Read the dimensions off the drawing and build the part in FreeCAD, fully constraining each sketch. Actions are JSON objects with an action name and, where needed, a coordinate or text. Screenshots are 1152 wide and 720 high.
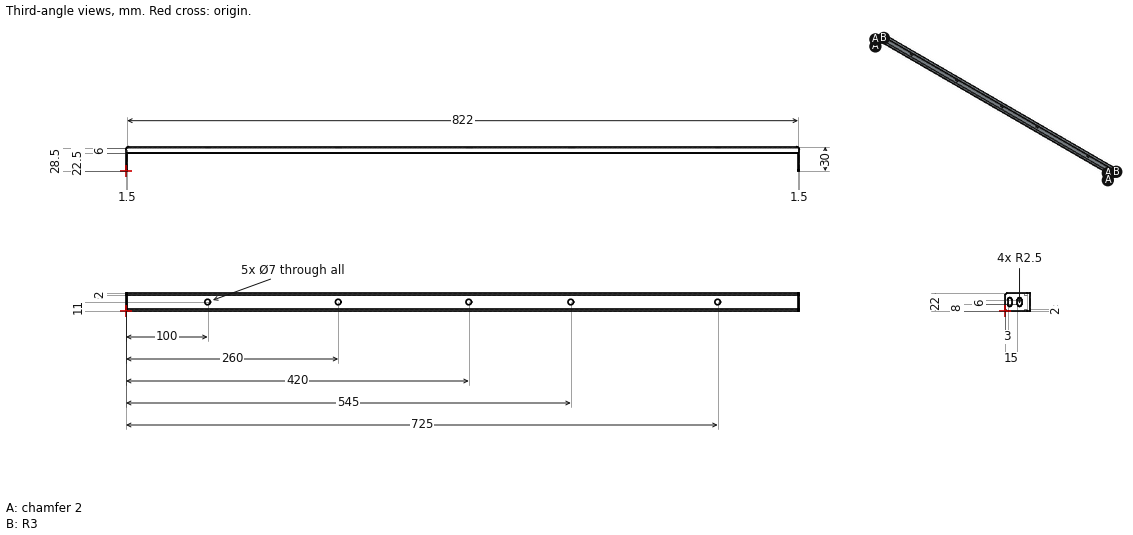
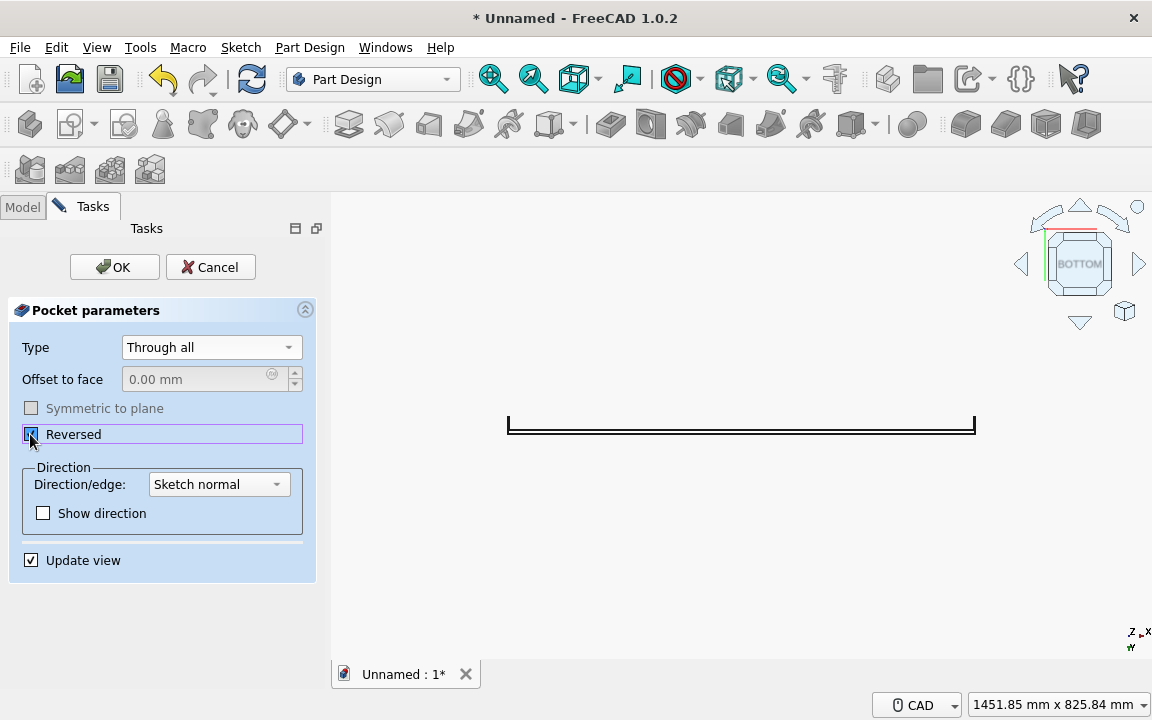
{"action": "left_click", "coordinate": [115, 267]}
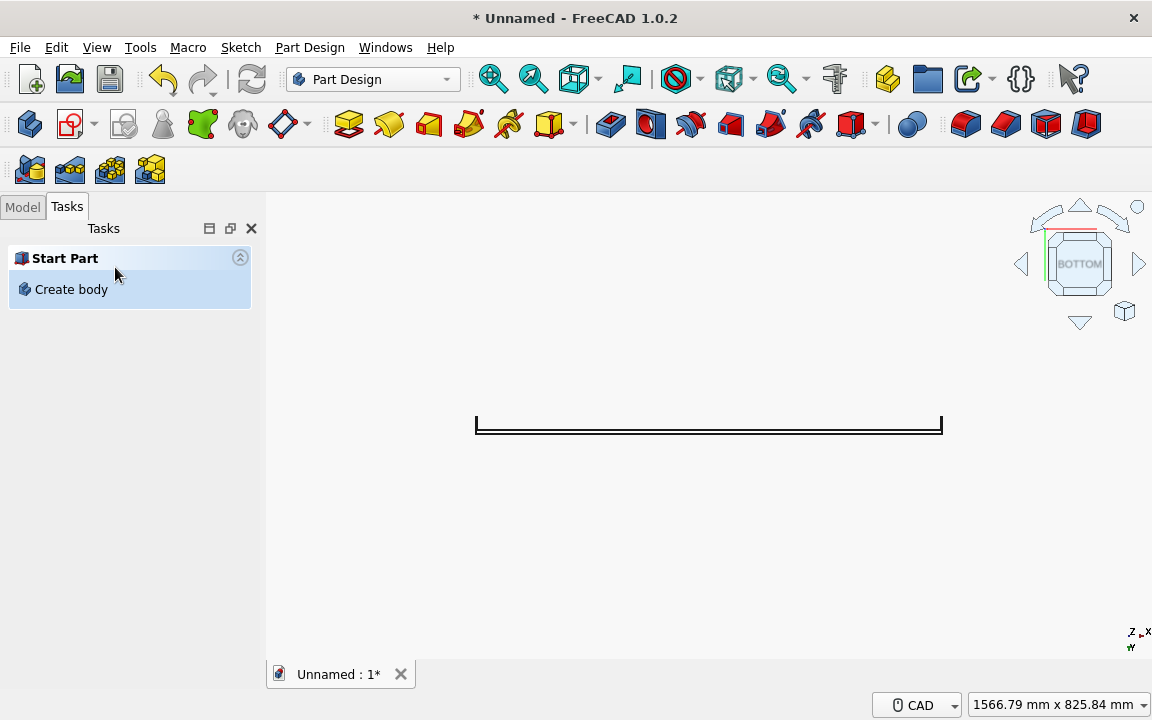
{"action": "scroll", "coordinate": [476, 416], "scroll_direction": "up", "scroll_amount": 15}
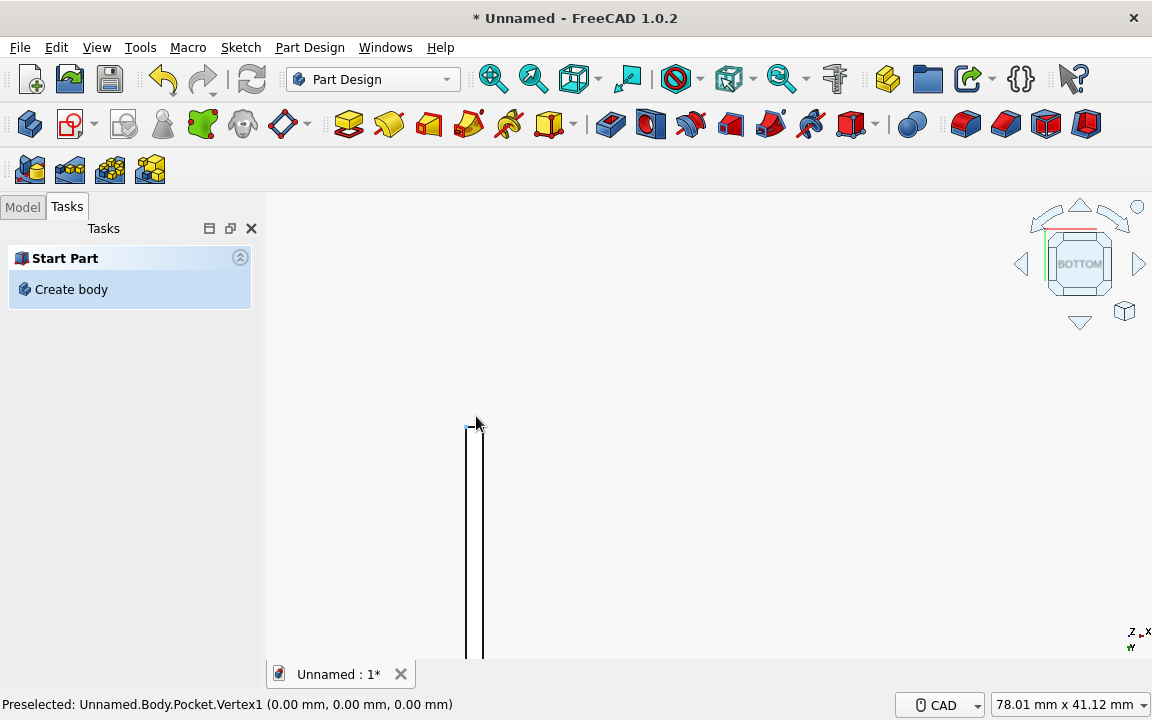
{"action": "scroll", "coordinate": [475, 426], "scroll_direction": "up", "scroll_amount": 5}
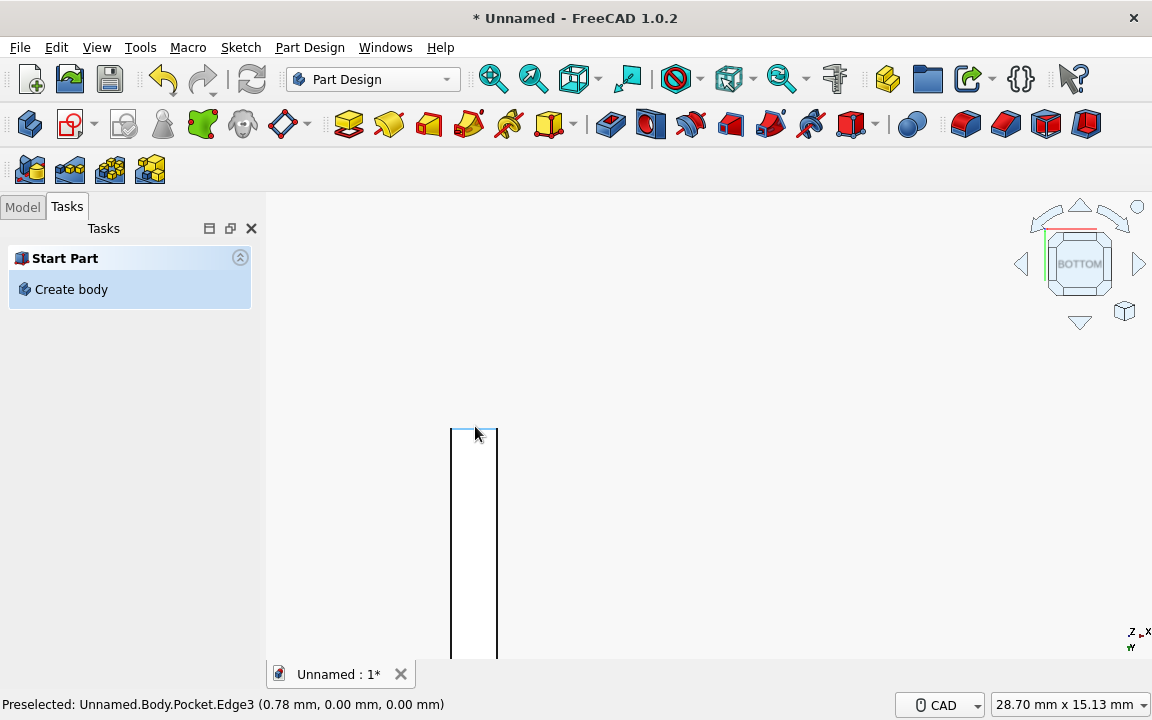
{"action": "left_click", "coordinate": [494, 80]}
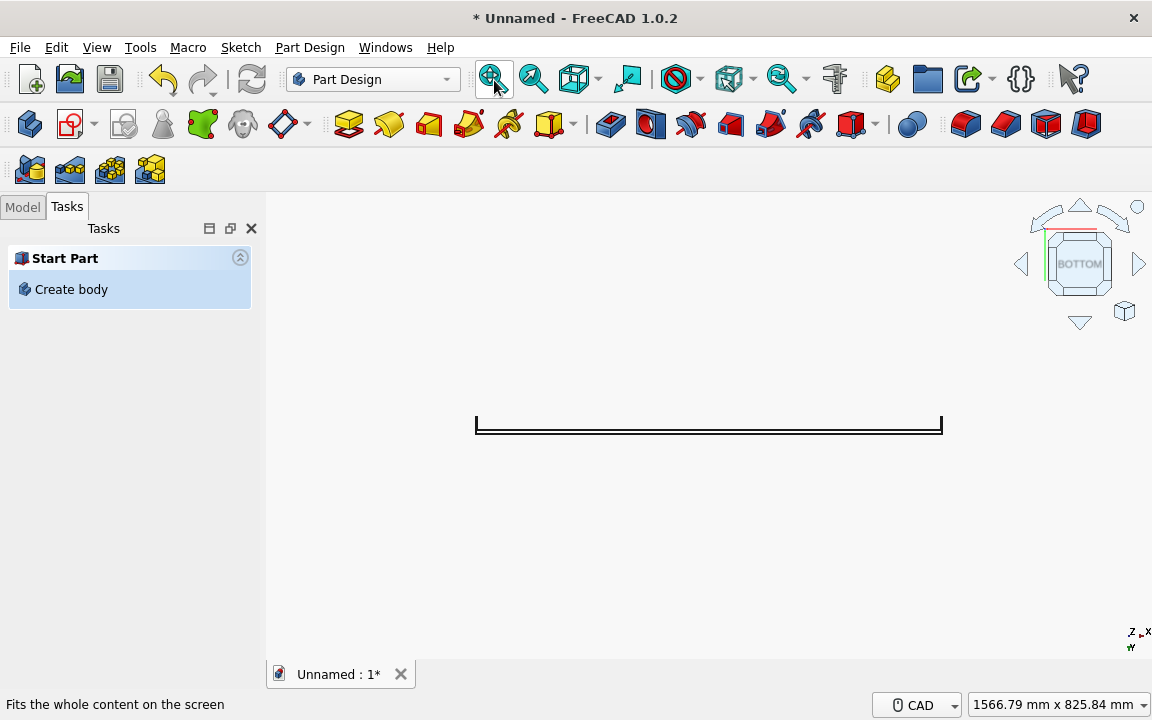
{"action": "key", "text": "0"}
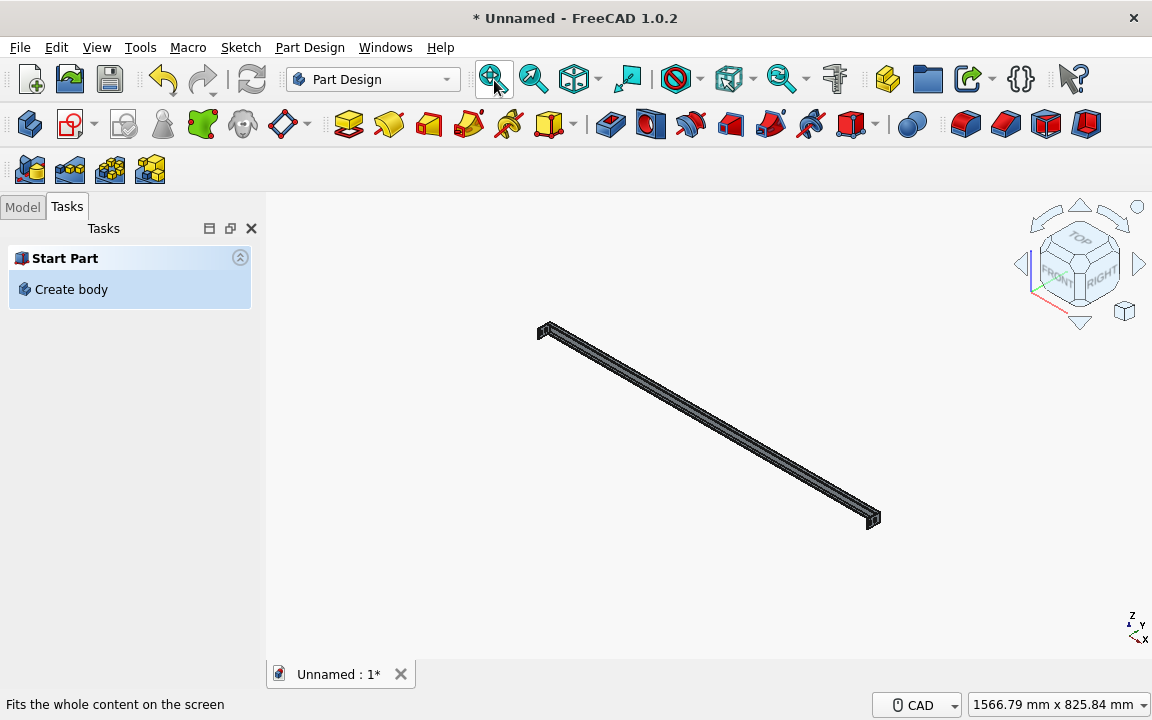
{"action": "left_click", "coordinate": [494, 80]}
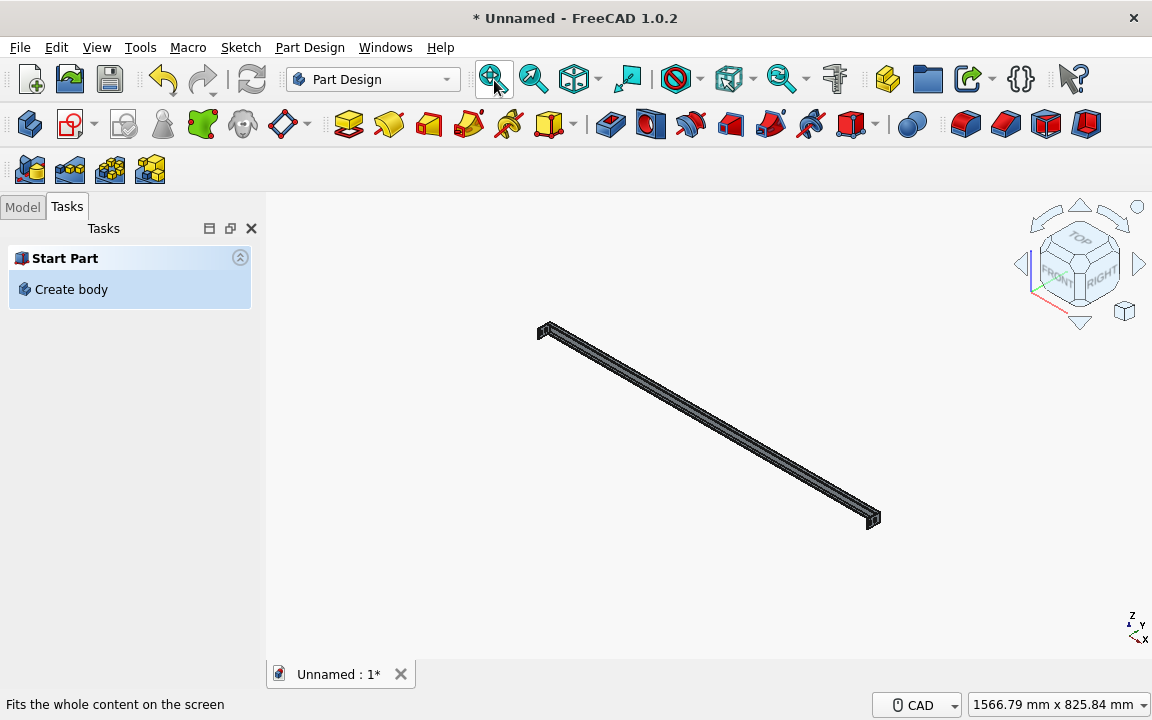
{"action": "scroll", "coordinate": [538, 338], "scroll_direction": "up", "scroll_amount": 15}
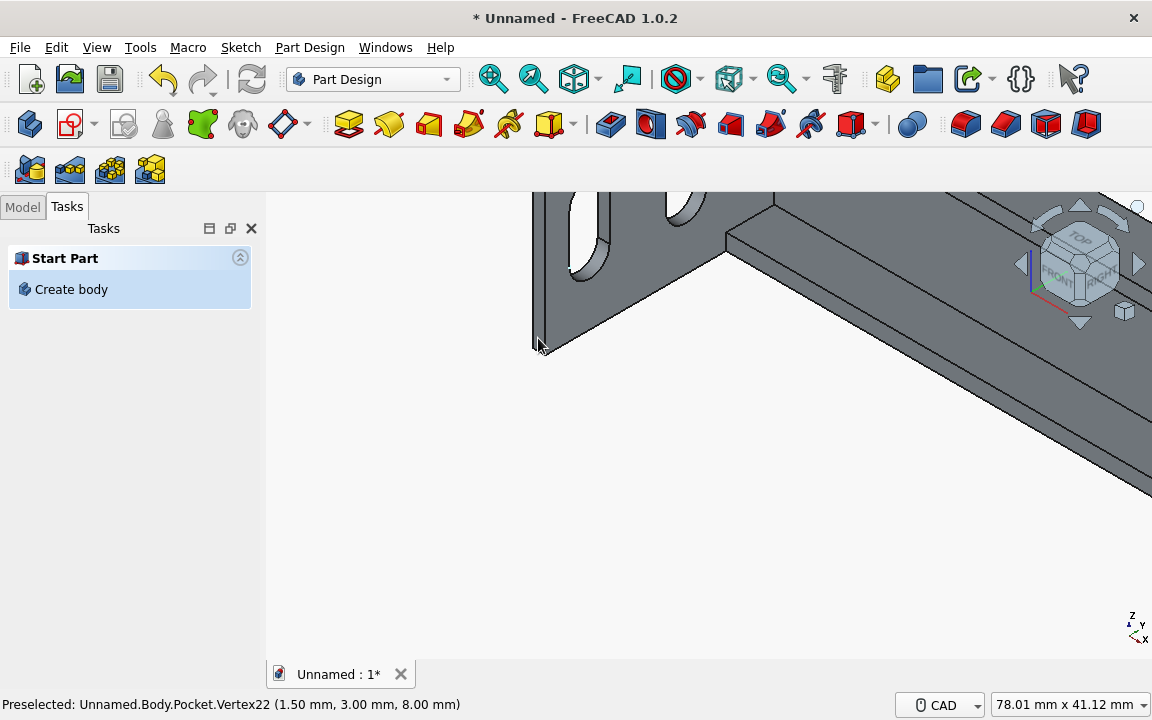
{"action": "scroll", "coordinate": [539, 351], "scroll_direction": "up", "scroll_amount": 5}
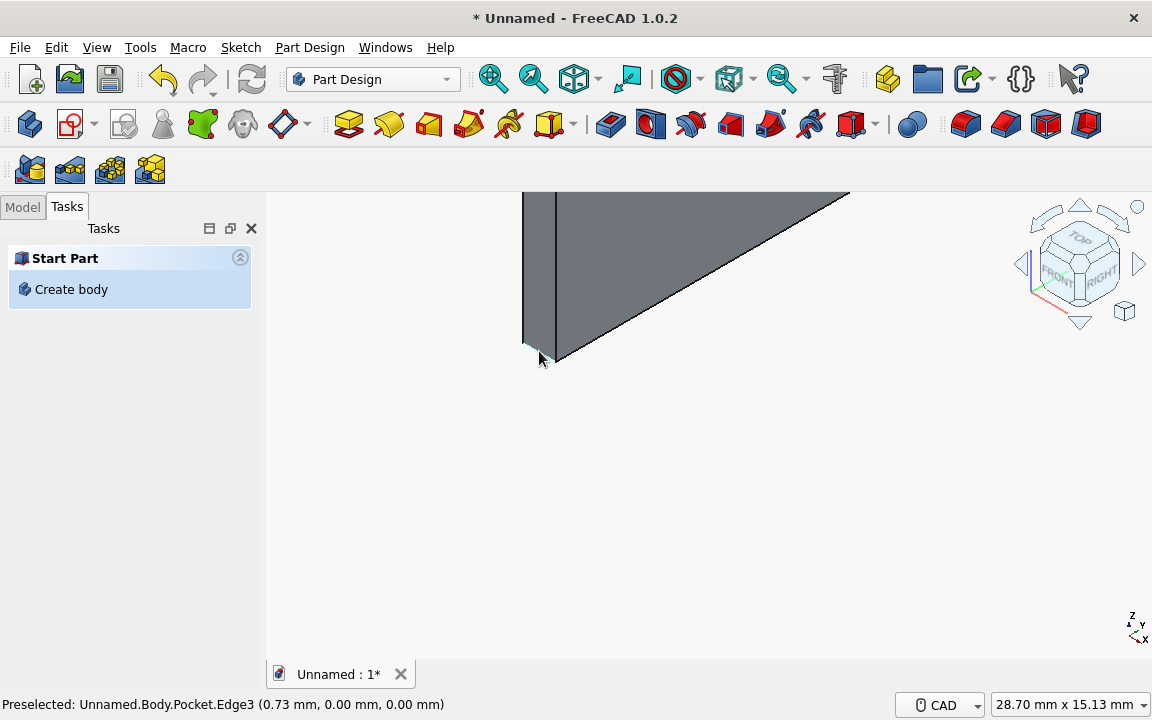
{"action": "left_click", "coordinate": [494, 80]}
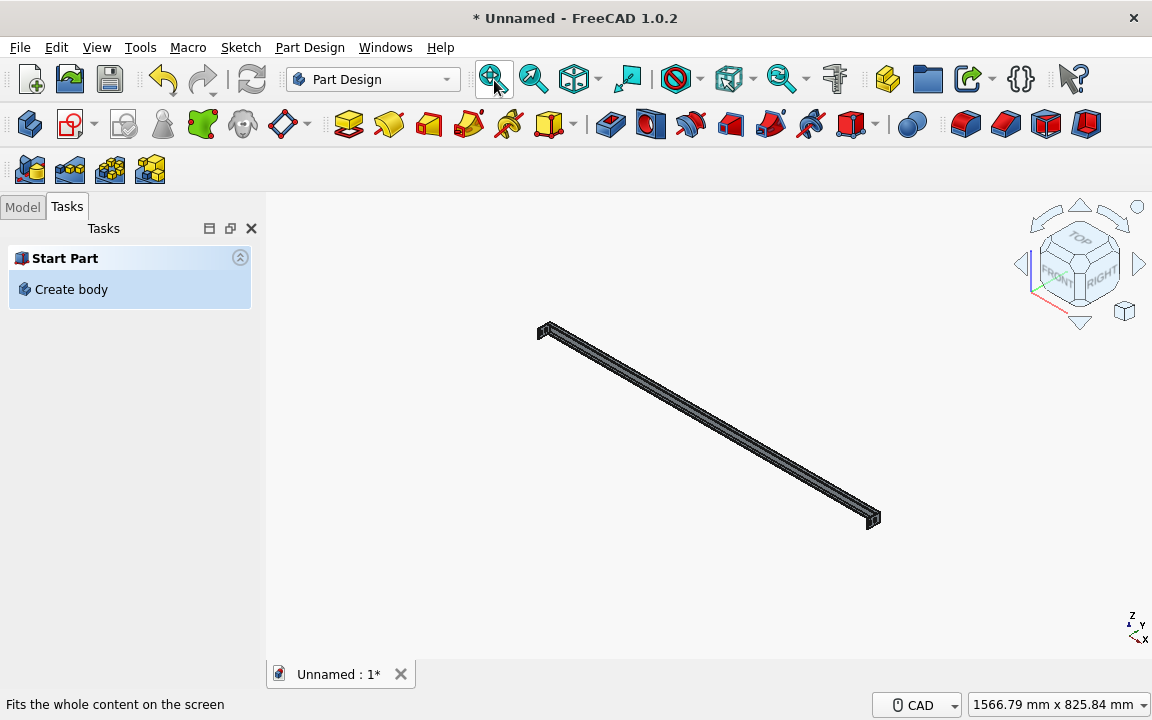
{"action": "key", "text": "2"}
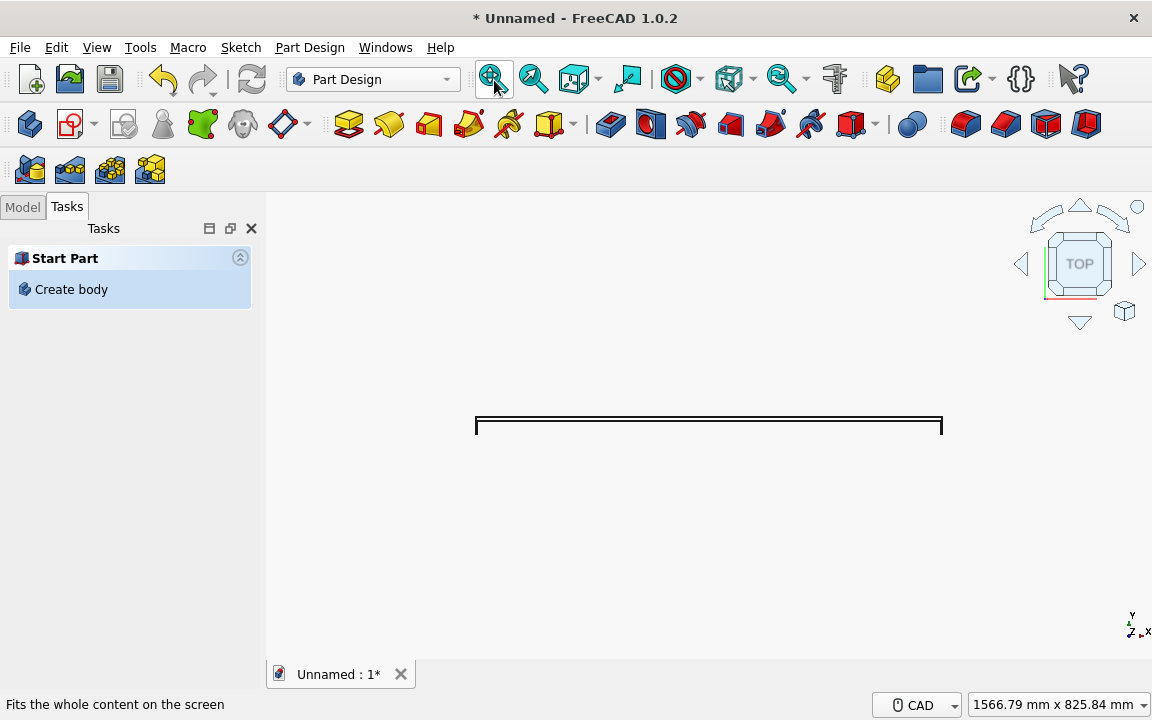
{"action": "scroll", "coordinate": [476, 433], "scroll_direction": "up", "scroll_amount": 15}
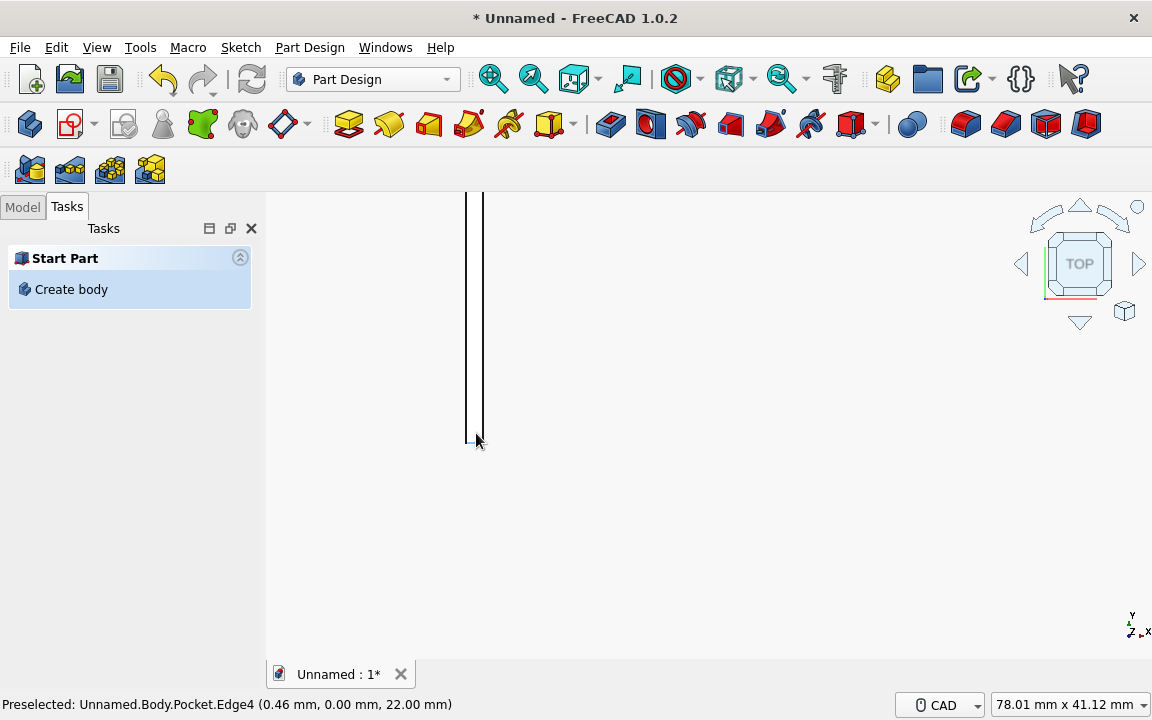
{"action": "left_click", "coordinate": [475, 442]}